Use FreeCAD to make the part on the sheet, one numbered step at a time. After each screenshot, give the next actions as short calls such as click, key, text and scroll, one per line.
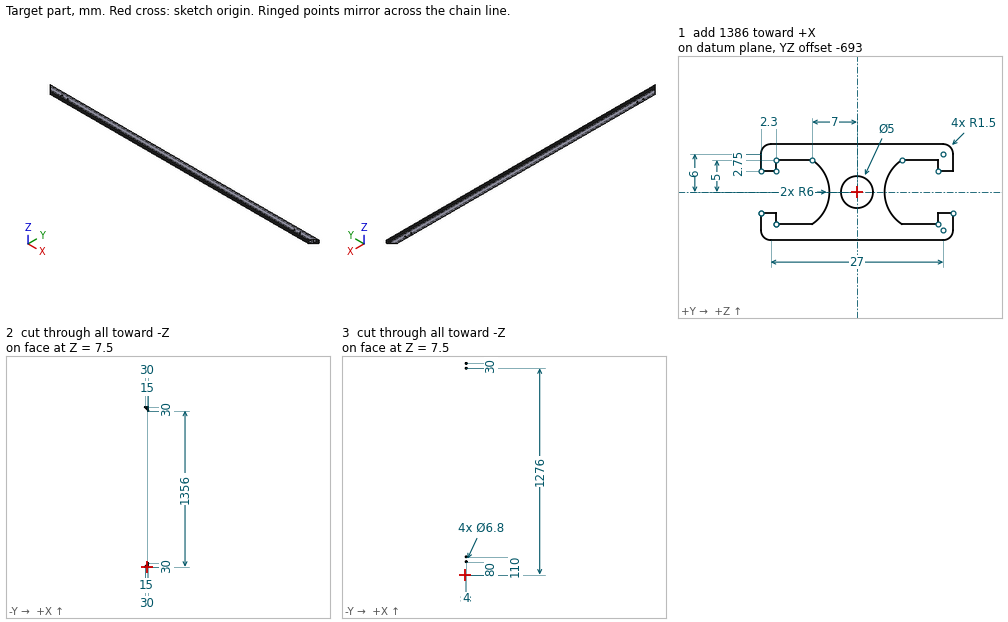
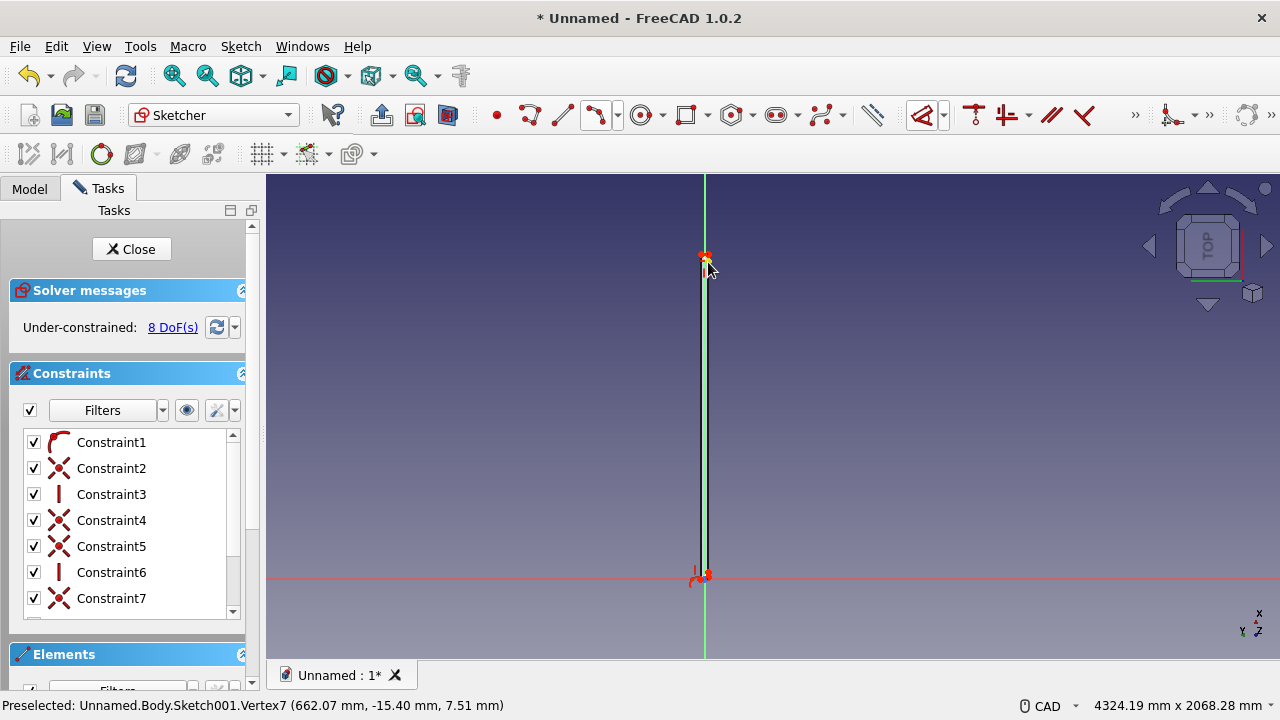
scroll(704, 579, up, 12)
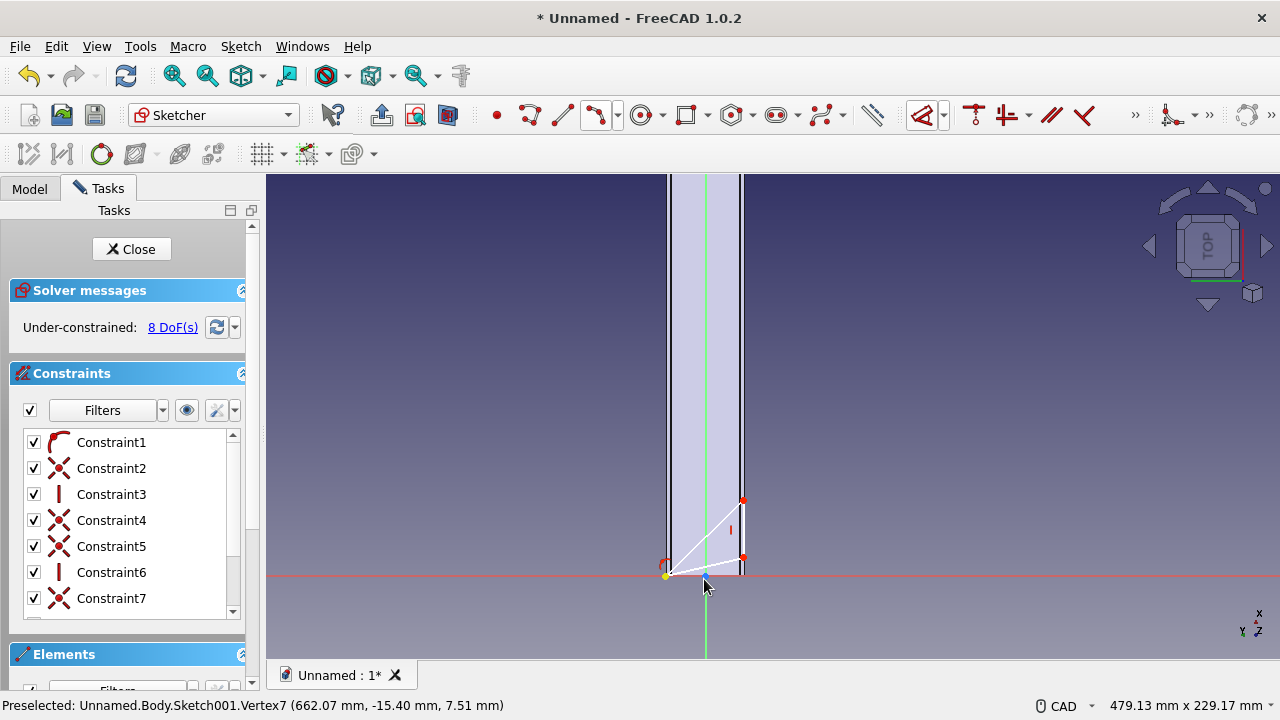
click(697, 569)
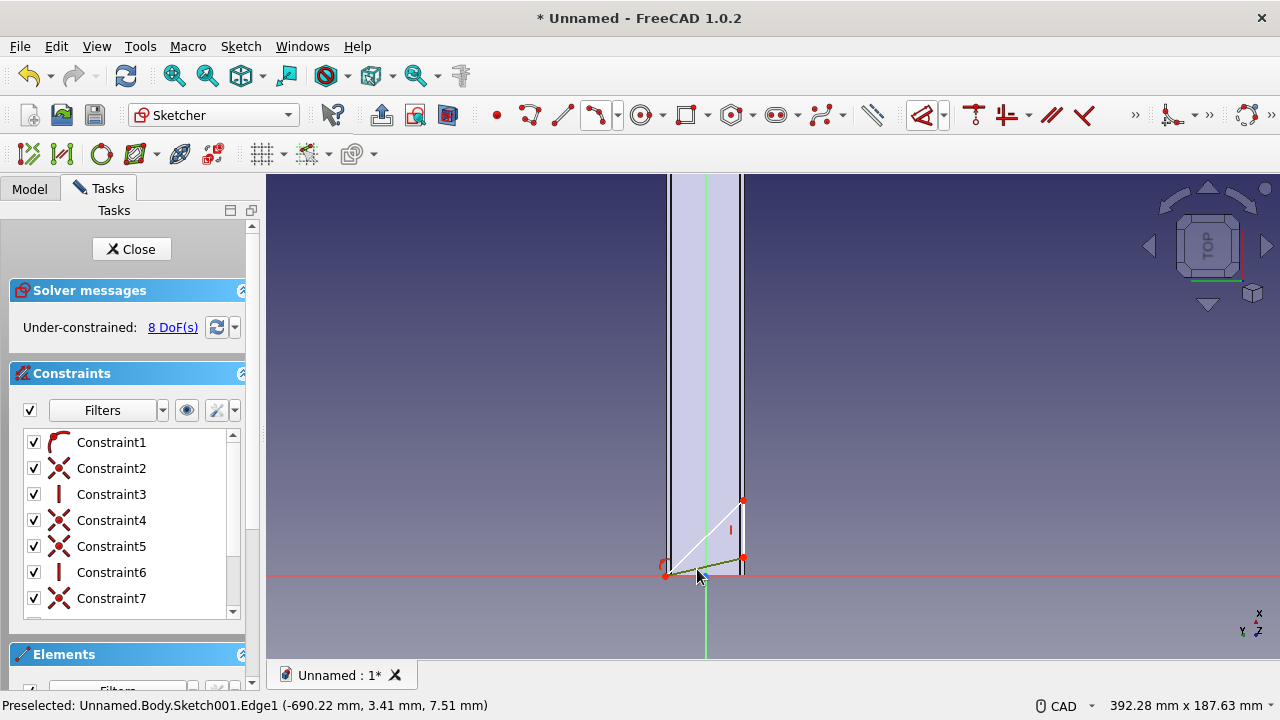
key(h)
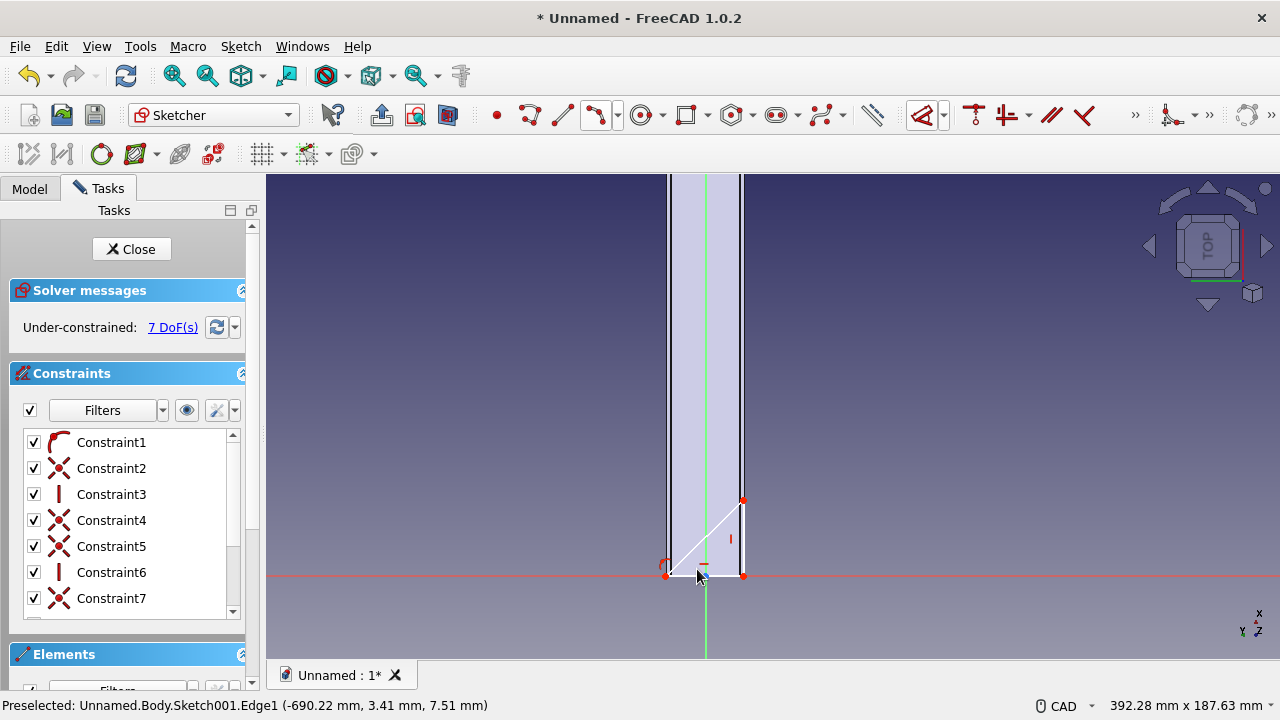
click(689, 576)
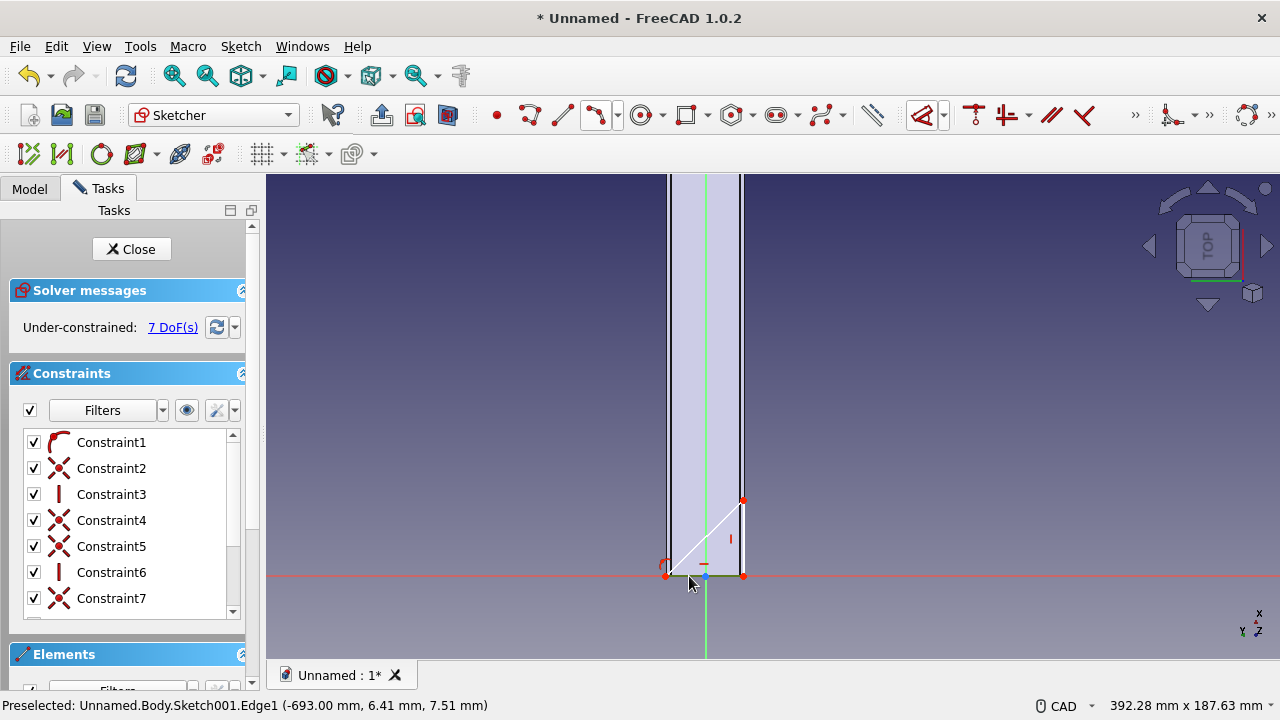
click(944, 116)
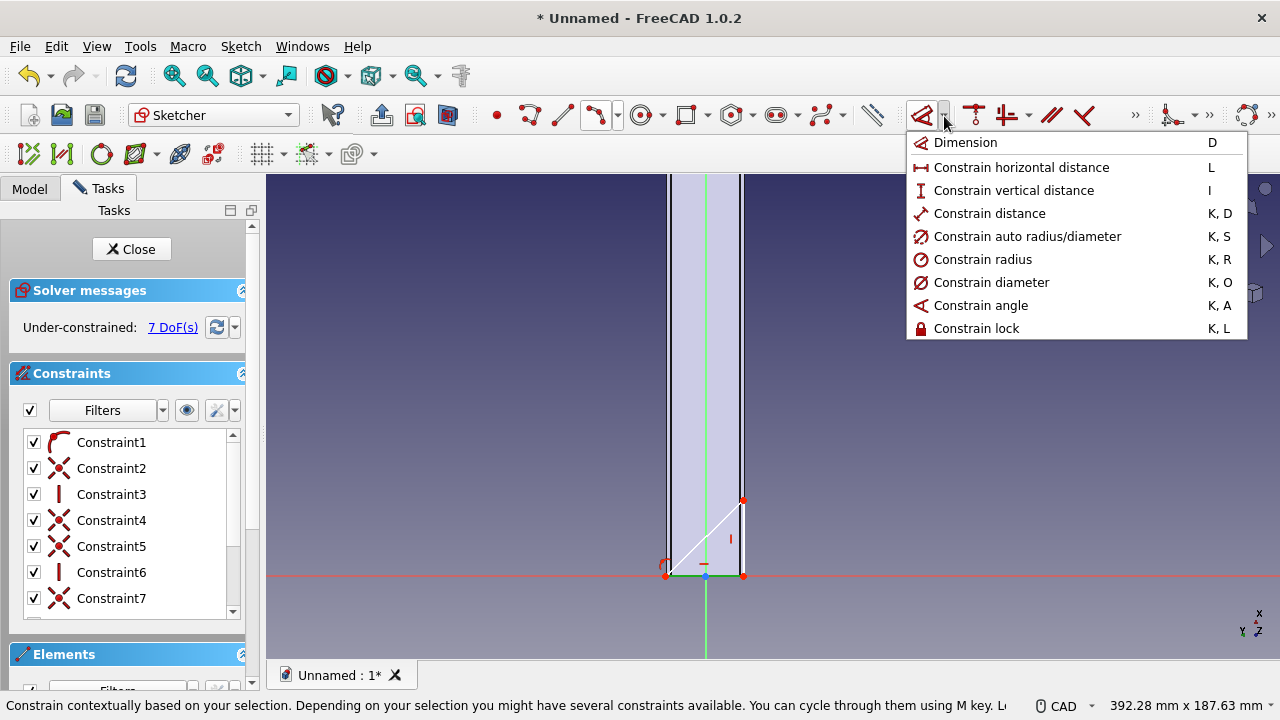
click(1077, 168)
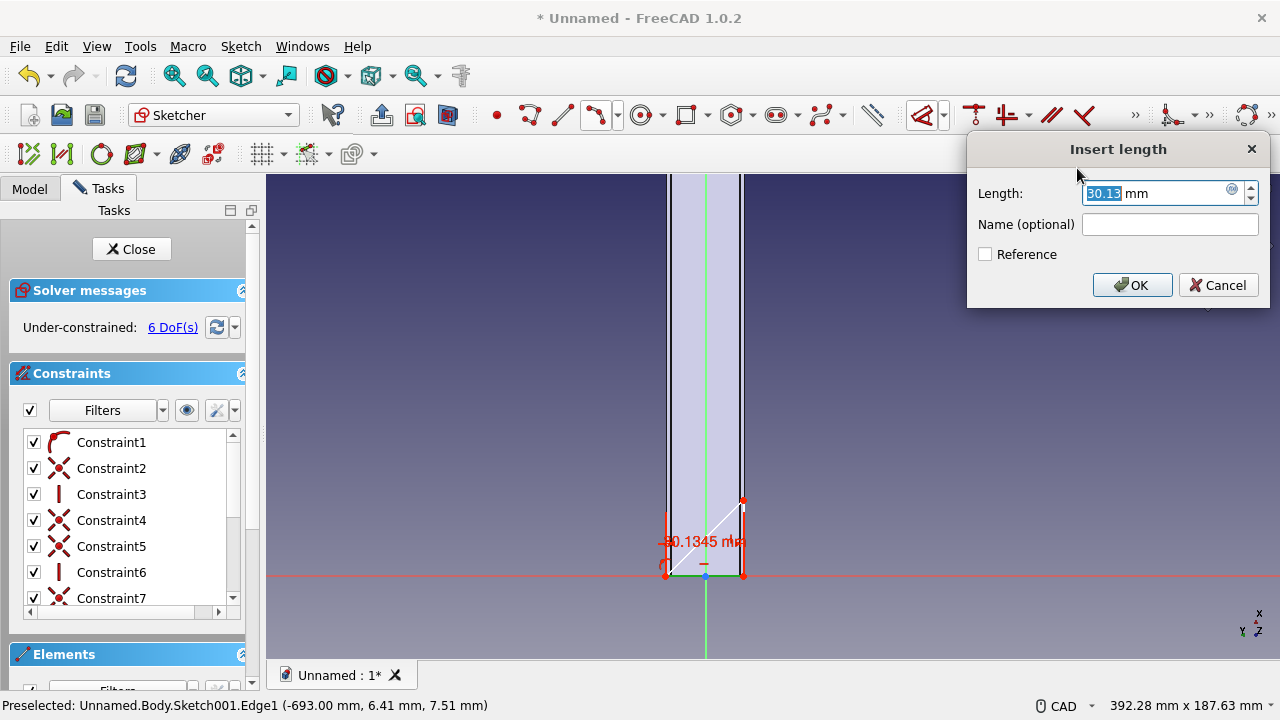
text(30)
key(Return)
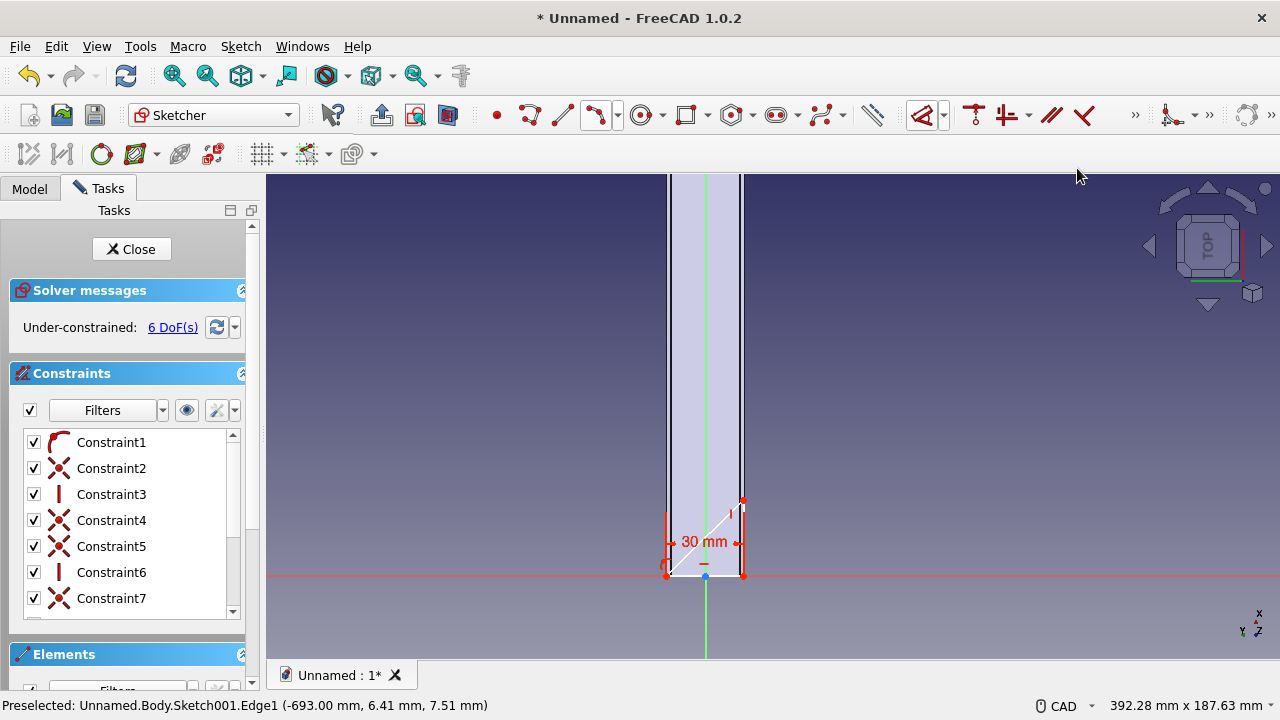
click(744, 553)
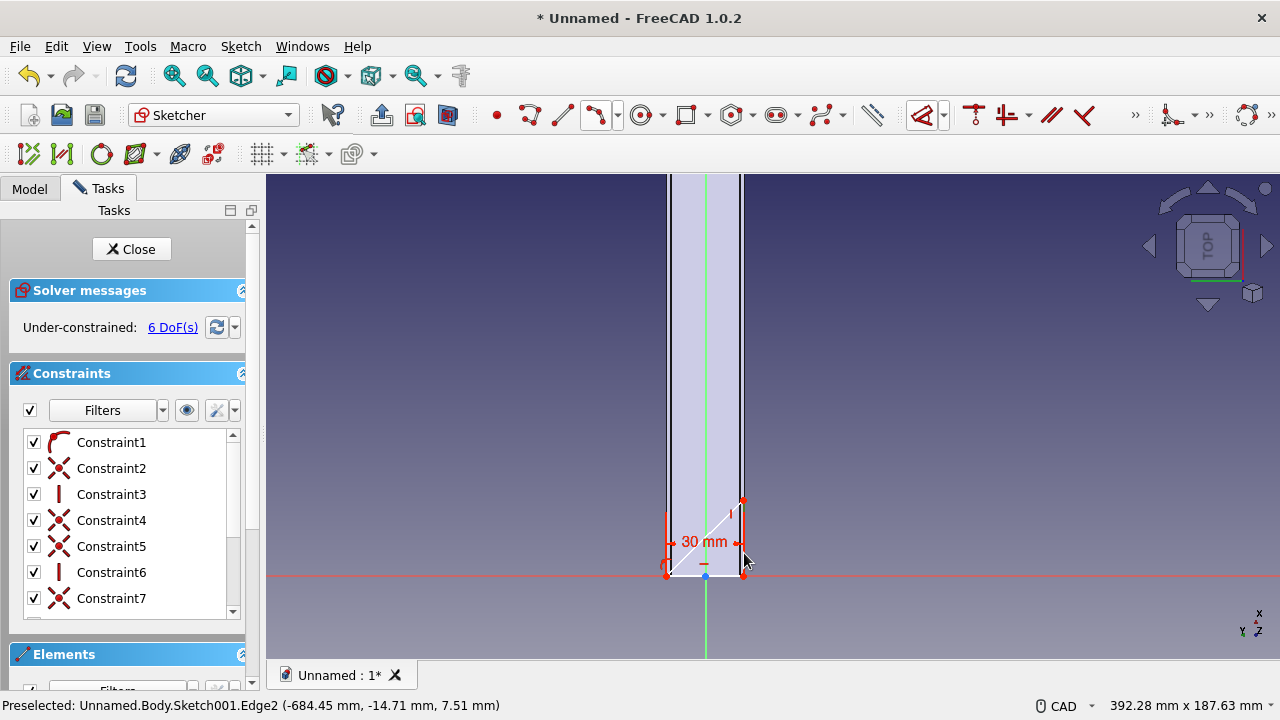
key(i)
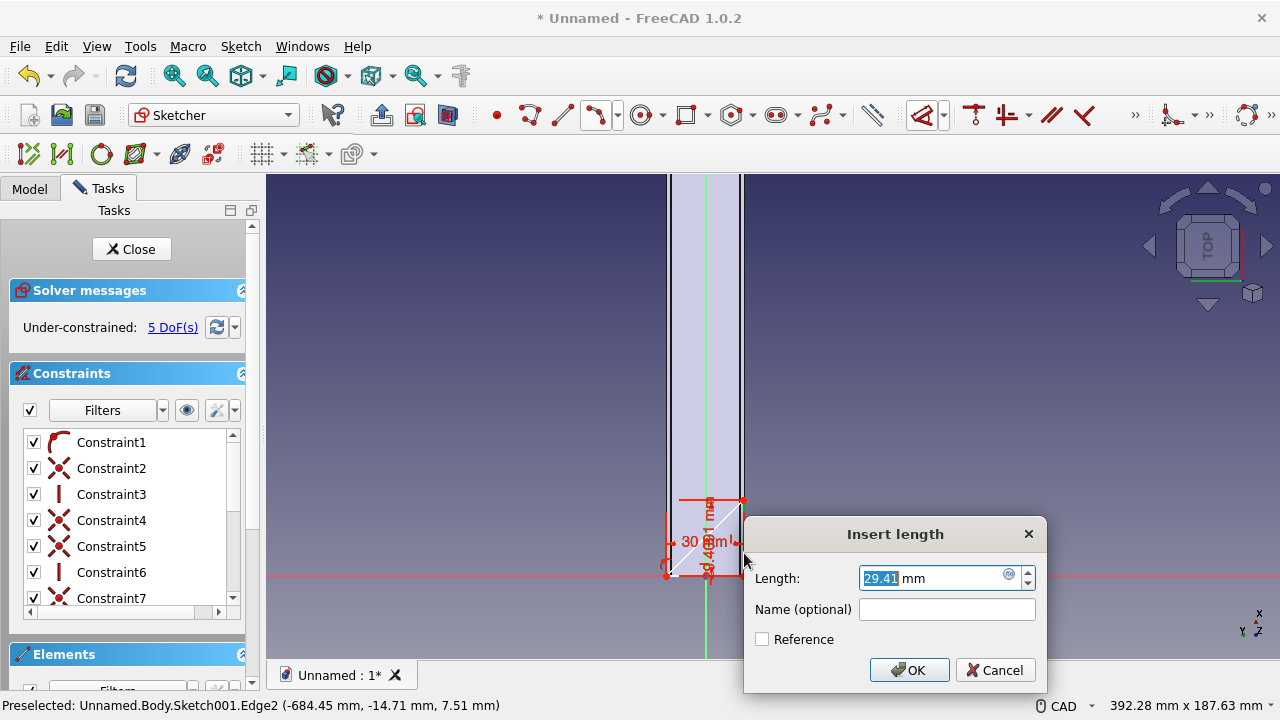
text(30)
key(Return)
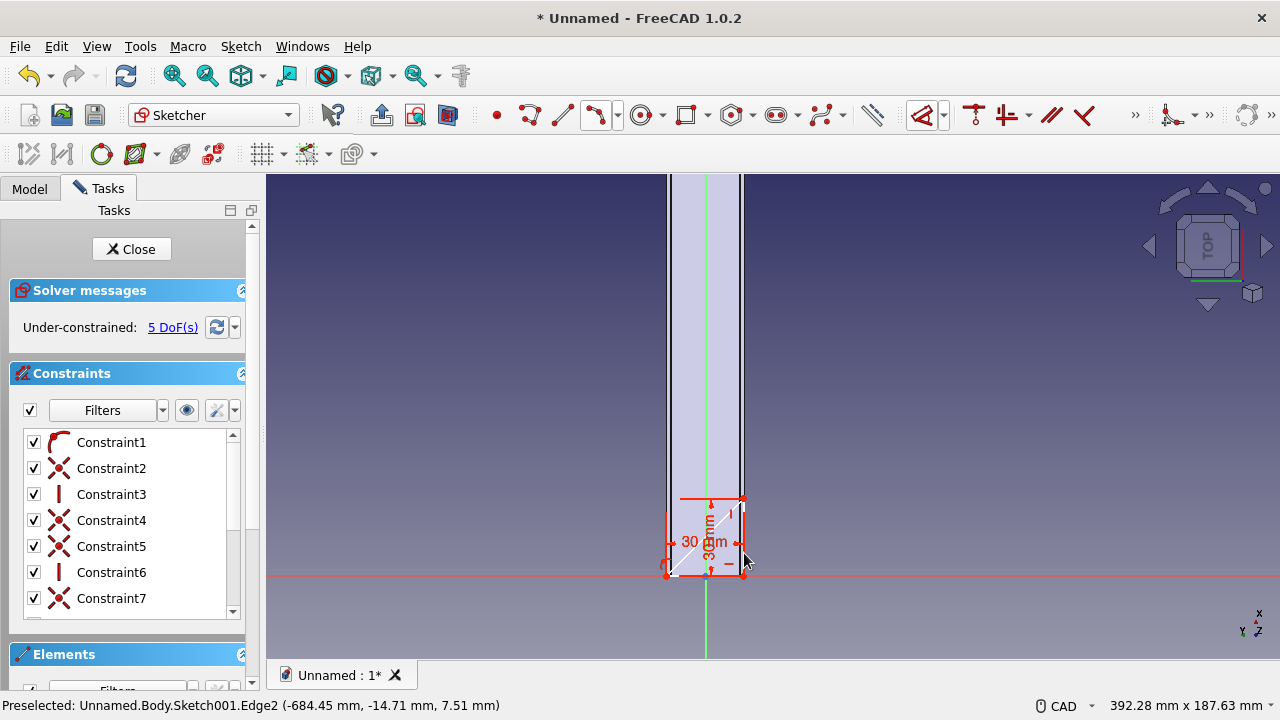
scroll(704, 579, down, 12)